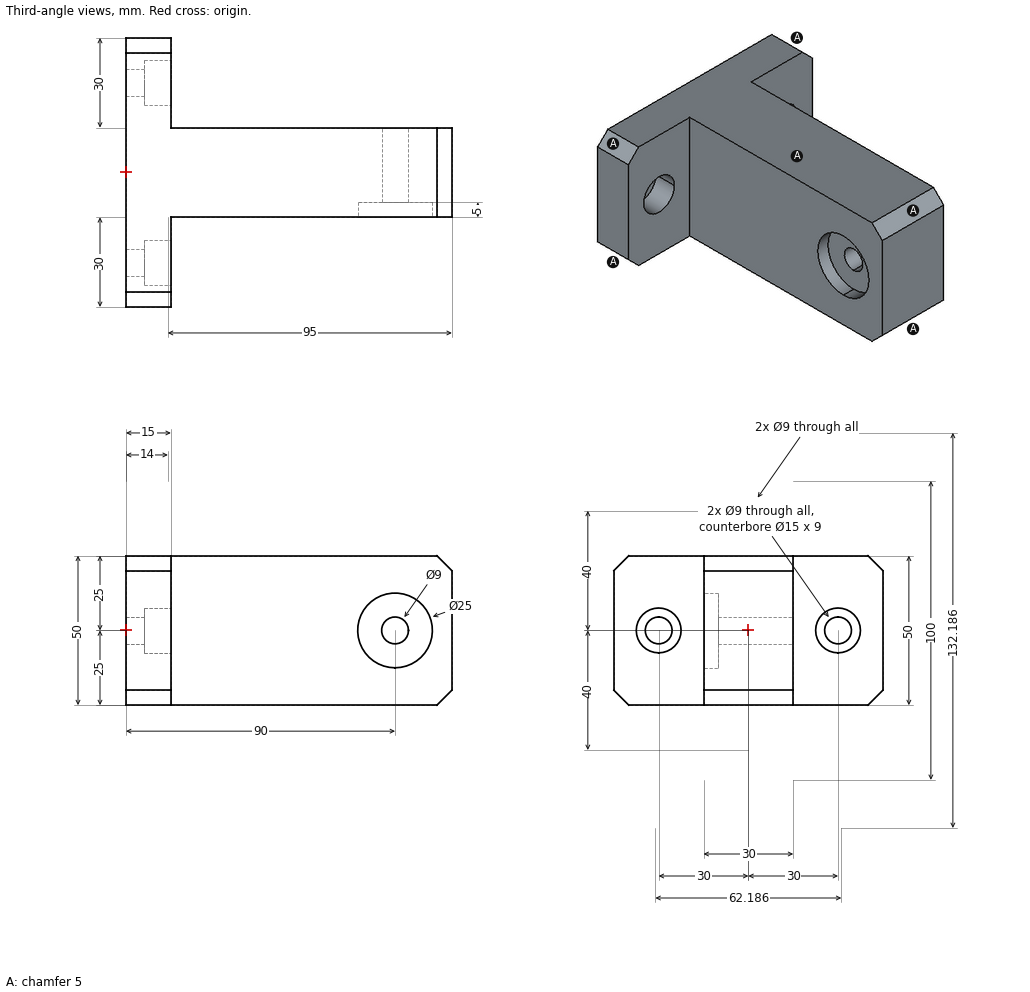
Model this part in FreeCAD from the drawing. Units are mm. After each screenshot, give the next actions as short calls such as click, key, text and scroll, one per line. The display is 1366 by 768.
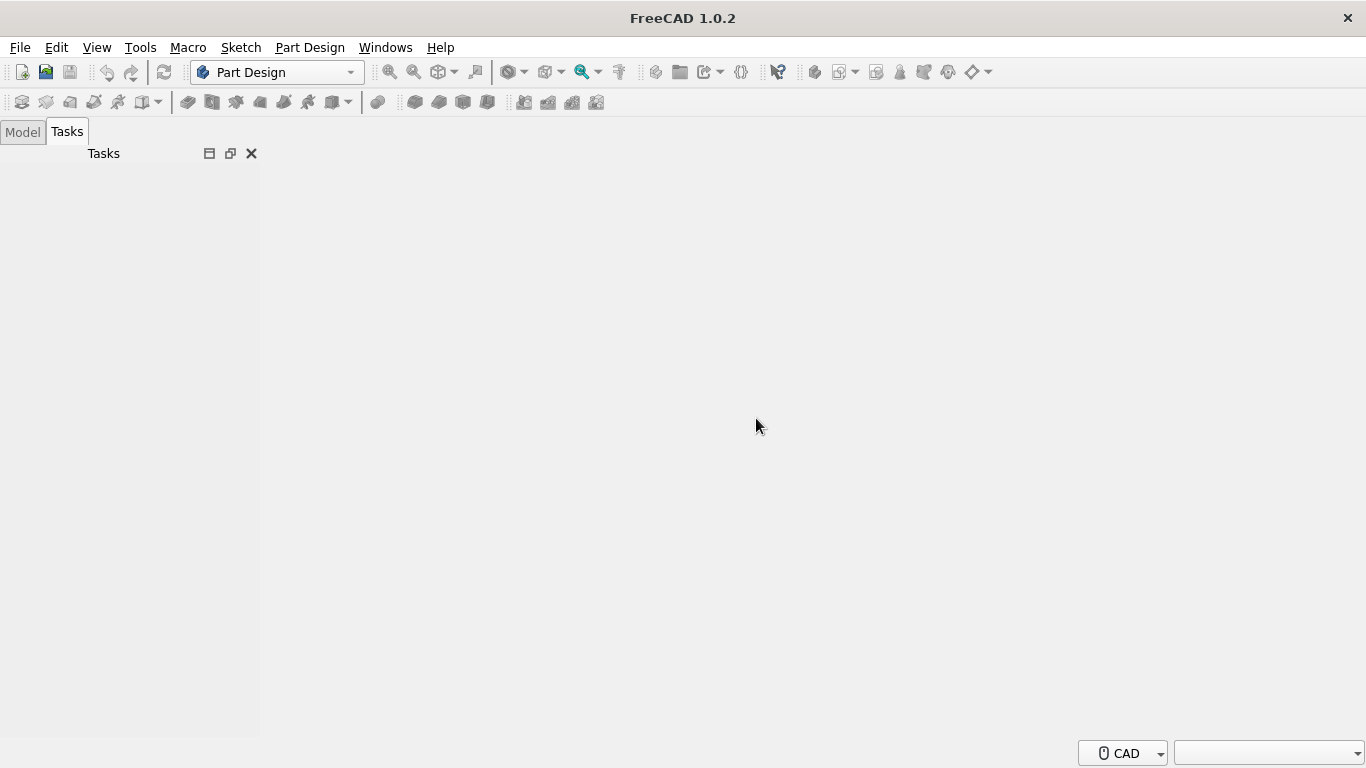
click(22, 72)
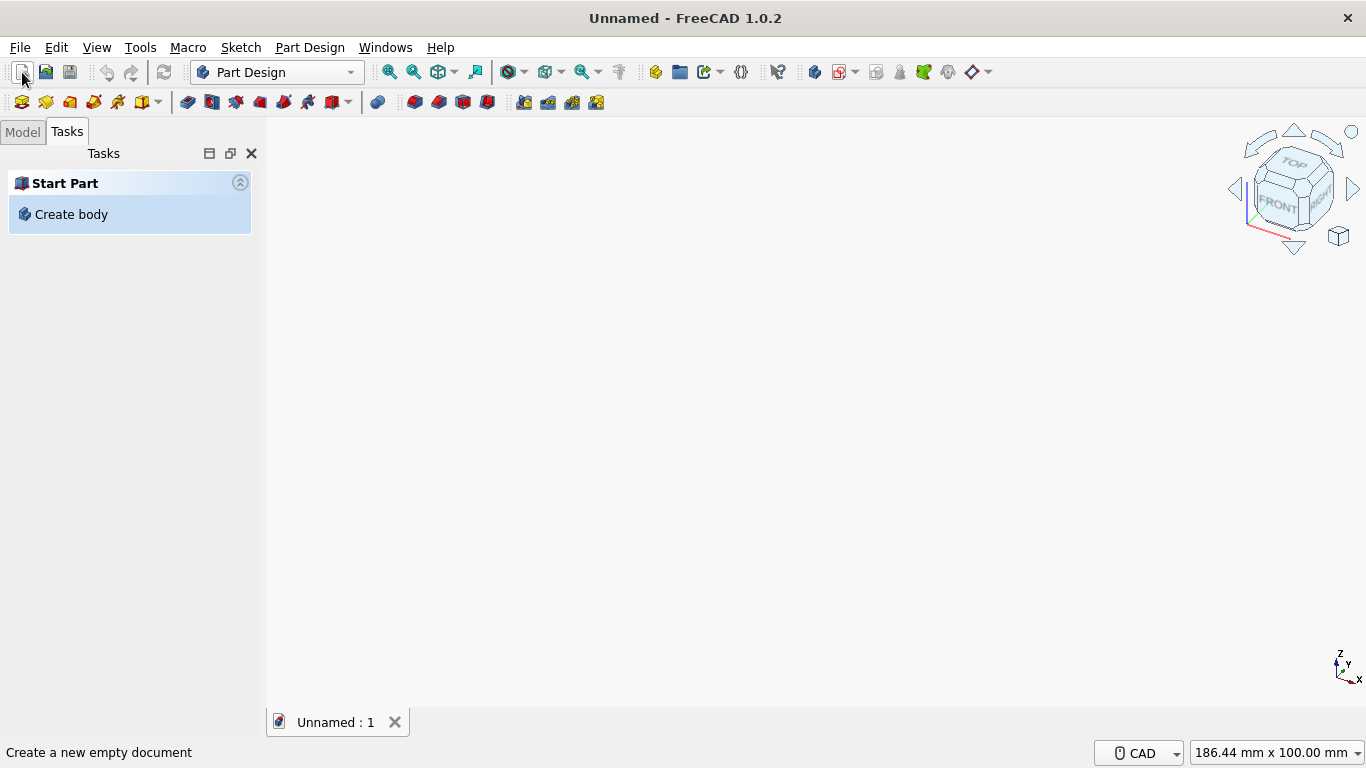
click(840, 72)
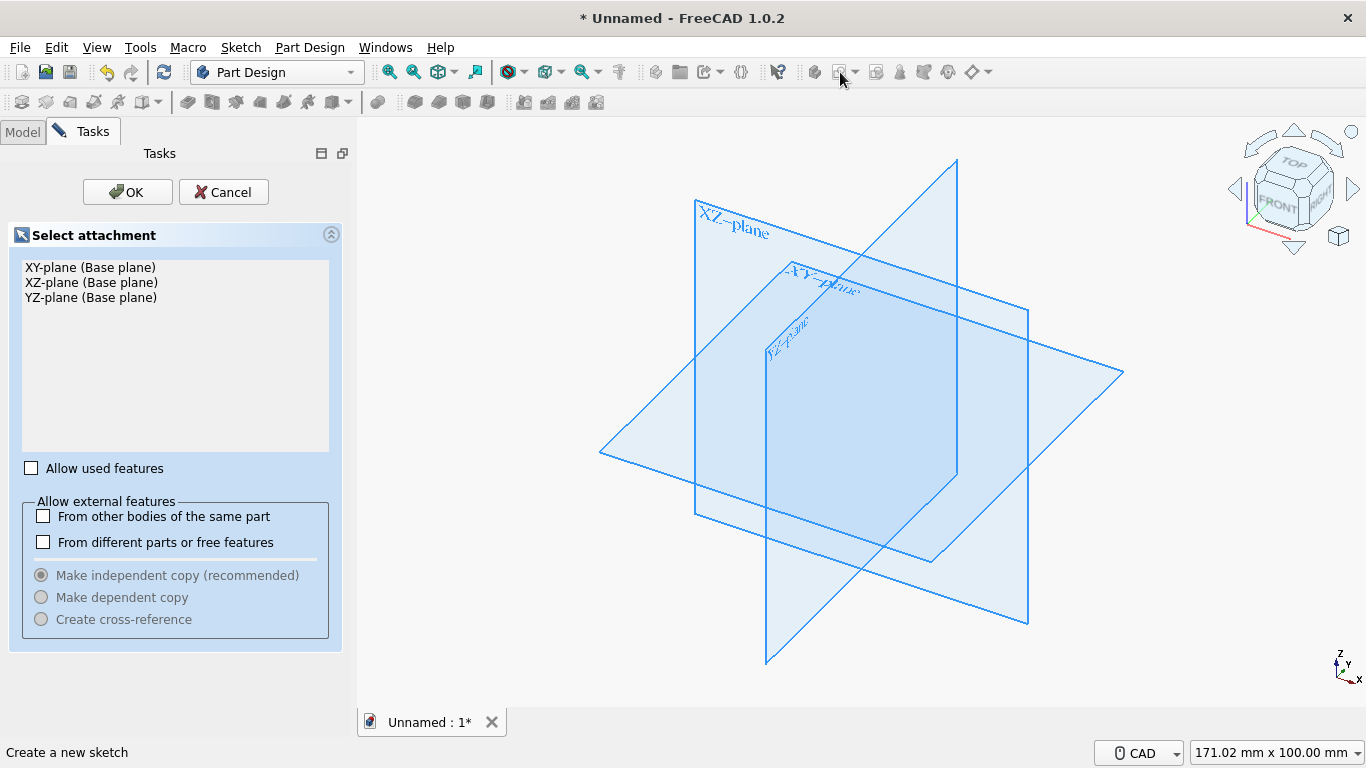
click(82, 298)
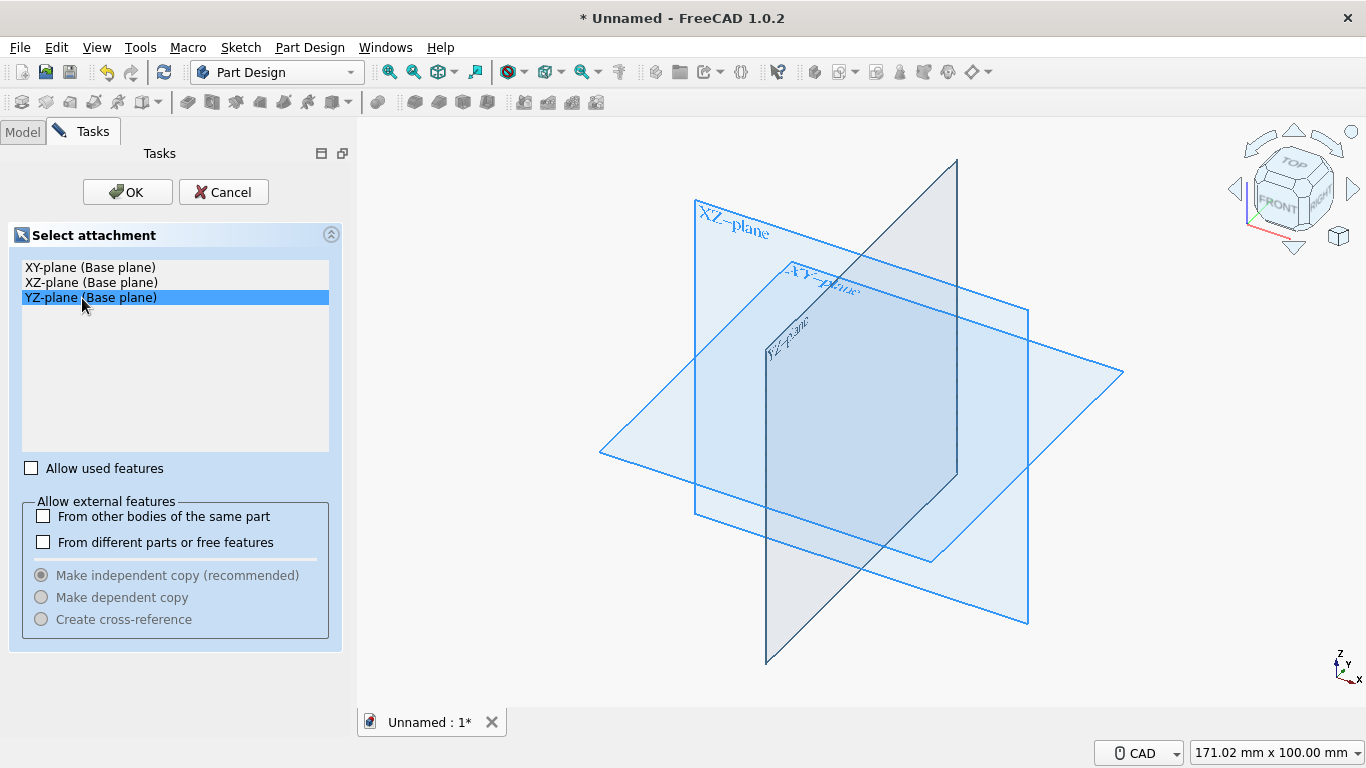
click(128, 192)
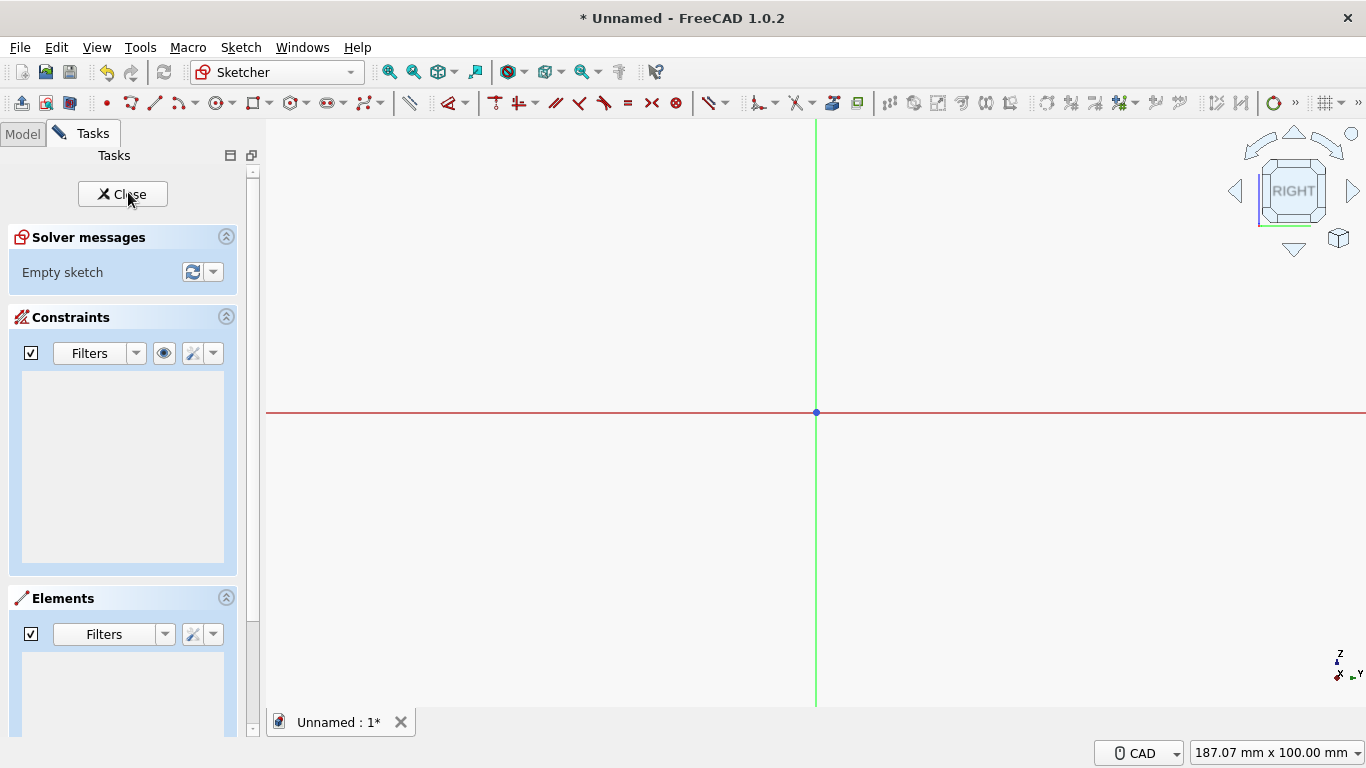
scroll(608, 413, down, 2)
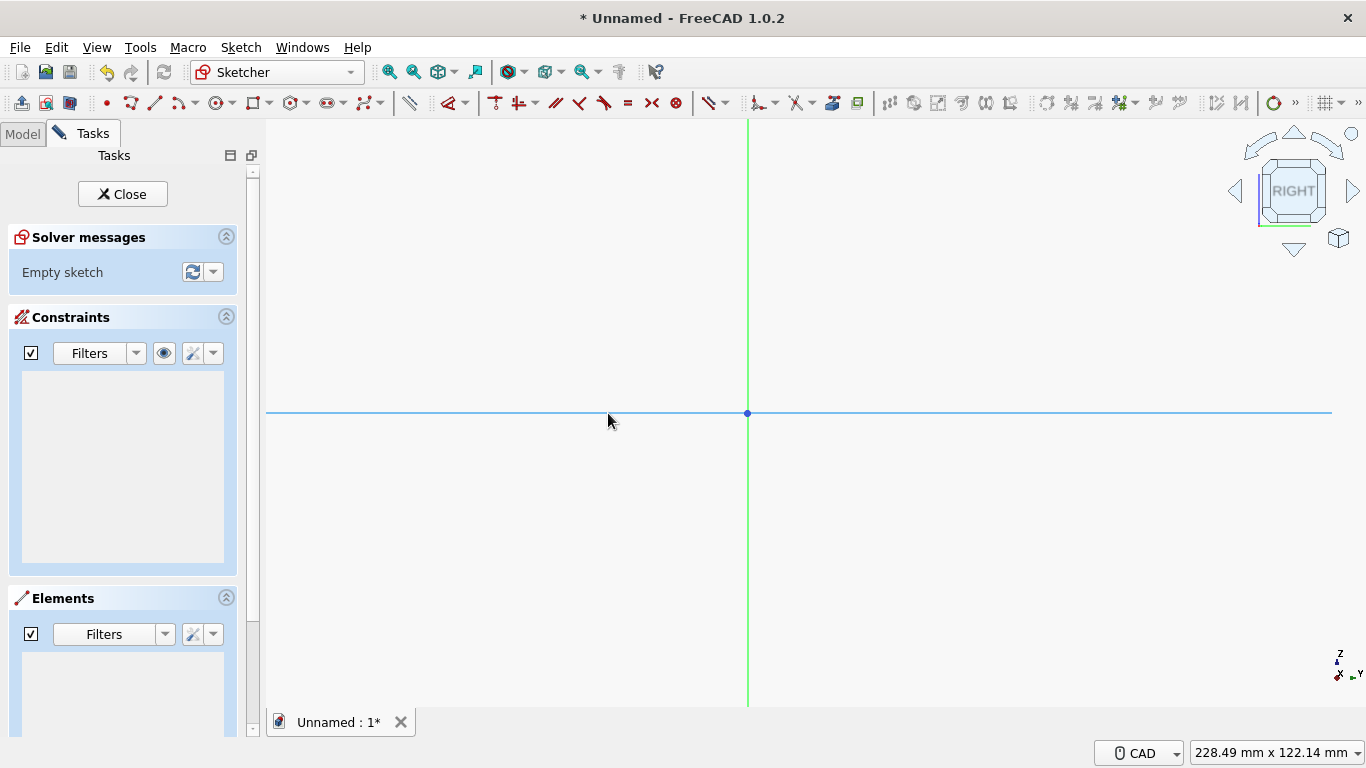
key(g)
key(v)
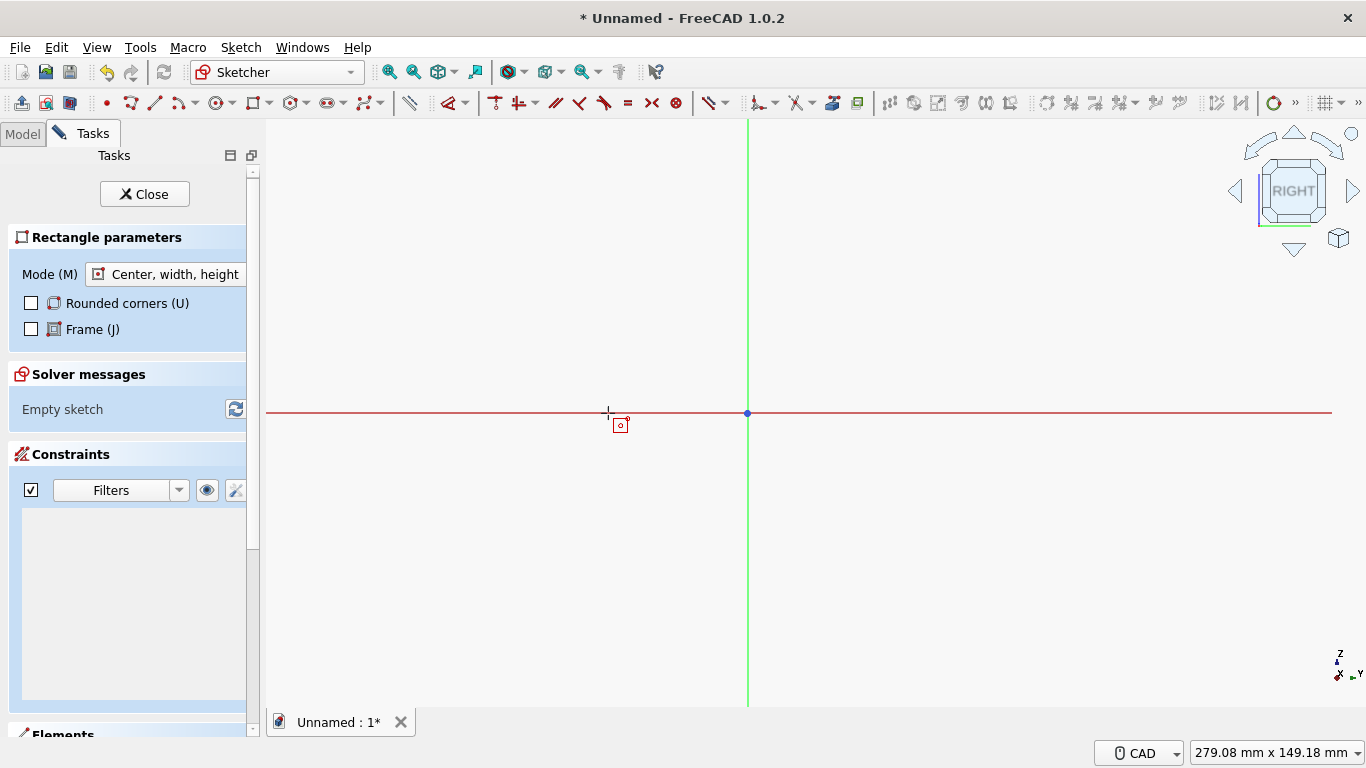
click(748, 413)
move(807, 216)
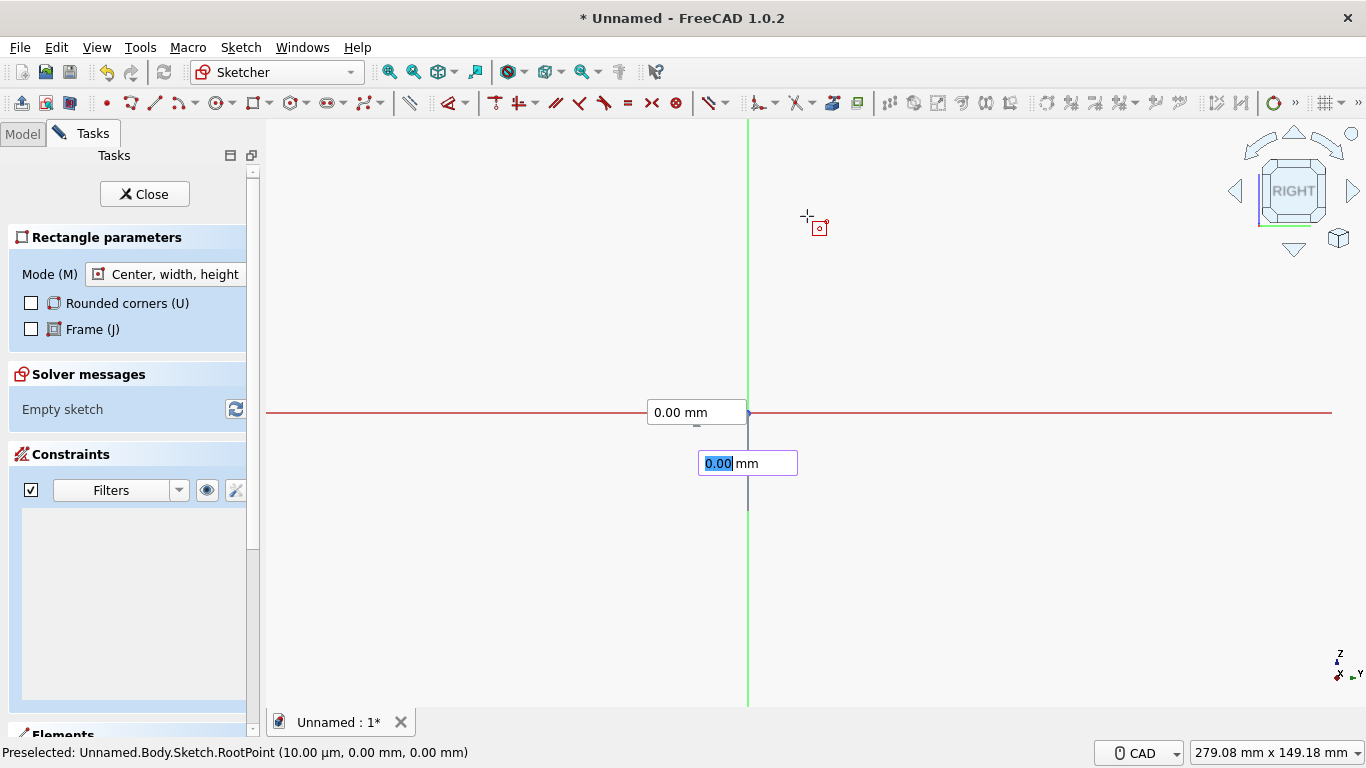
text(30)
key(Tab)
text(100)
key(Return)
key(Escape)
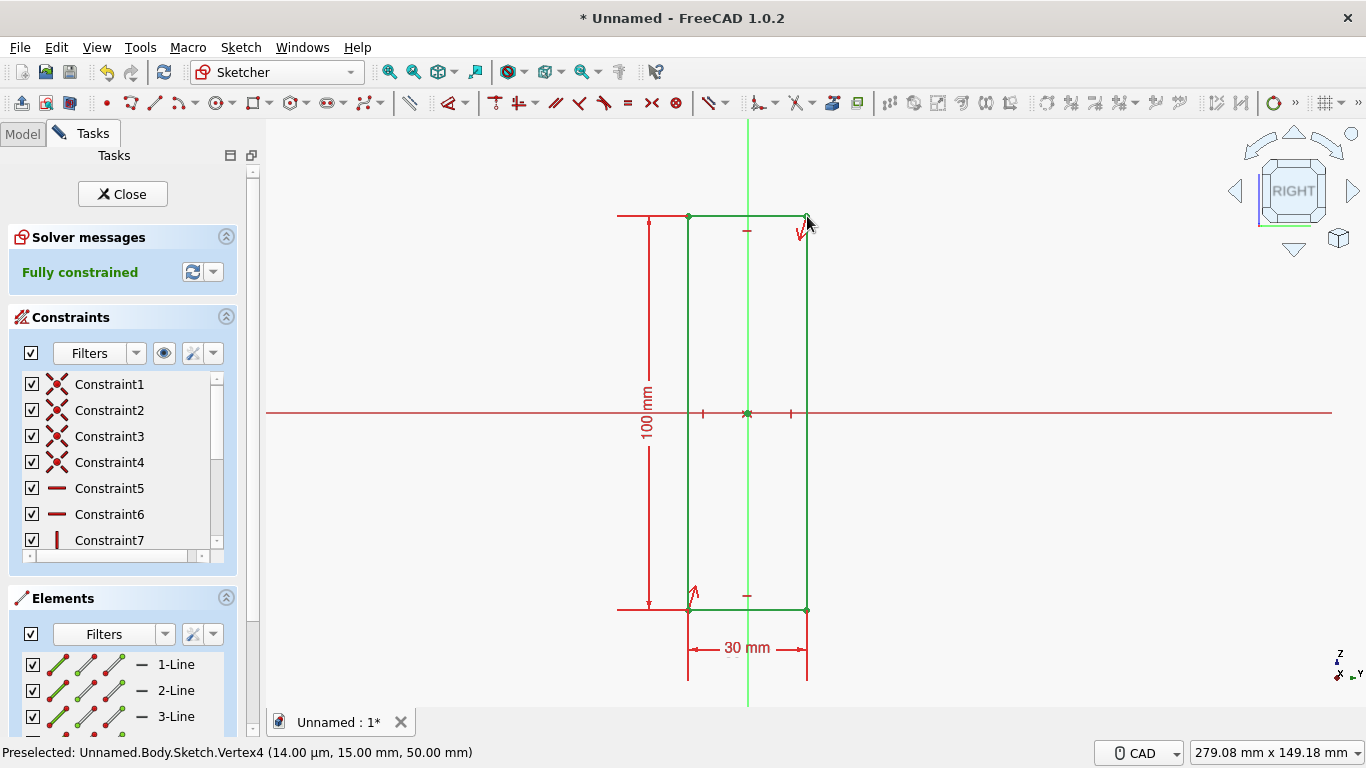
click(123, 194)